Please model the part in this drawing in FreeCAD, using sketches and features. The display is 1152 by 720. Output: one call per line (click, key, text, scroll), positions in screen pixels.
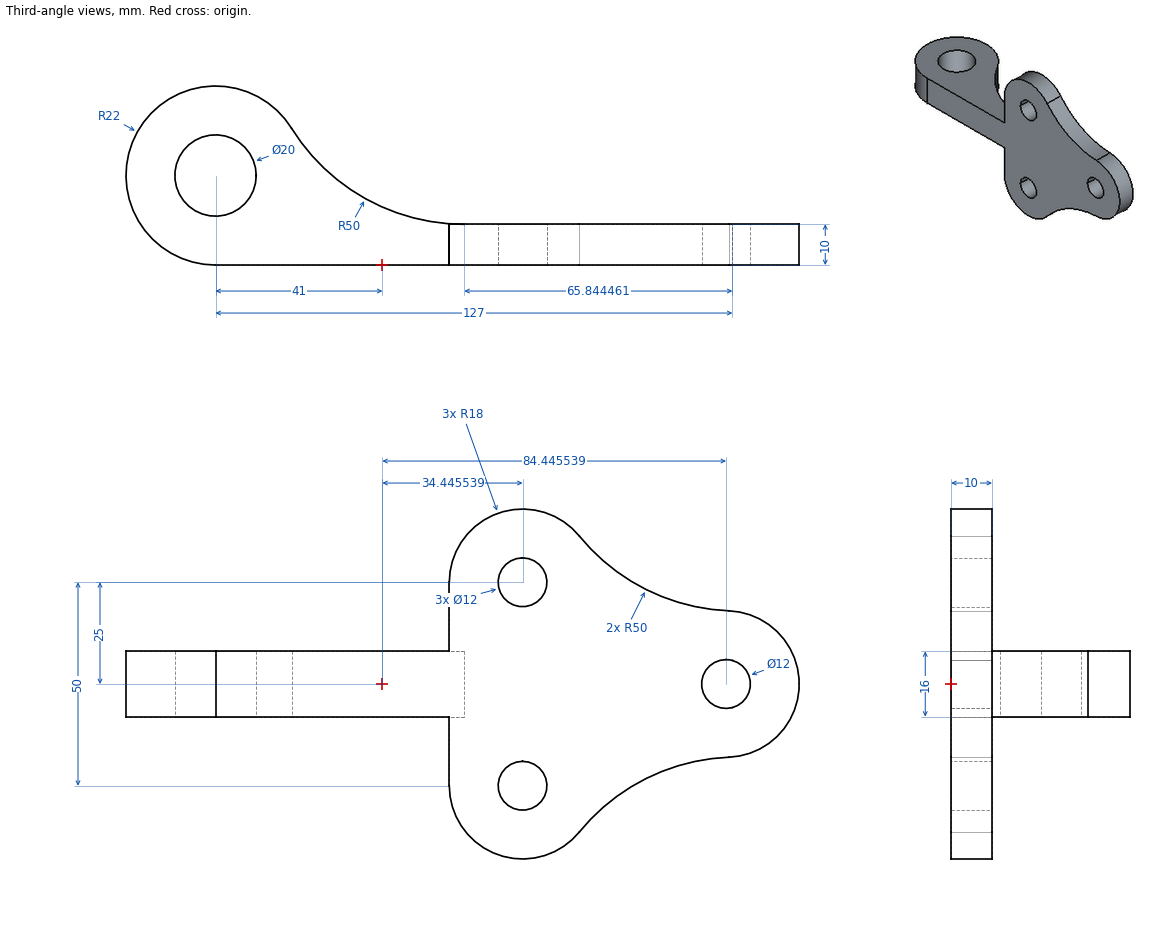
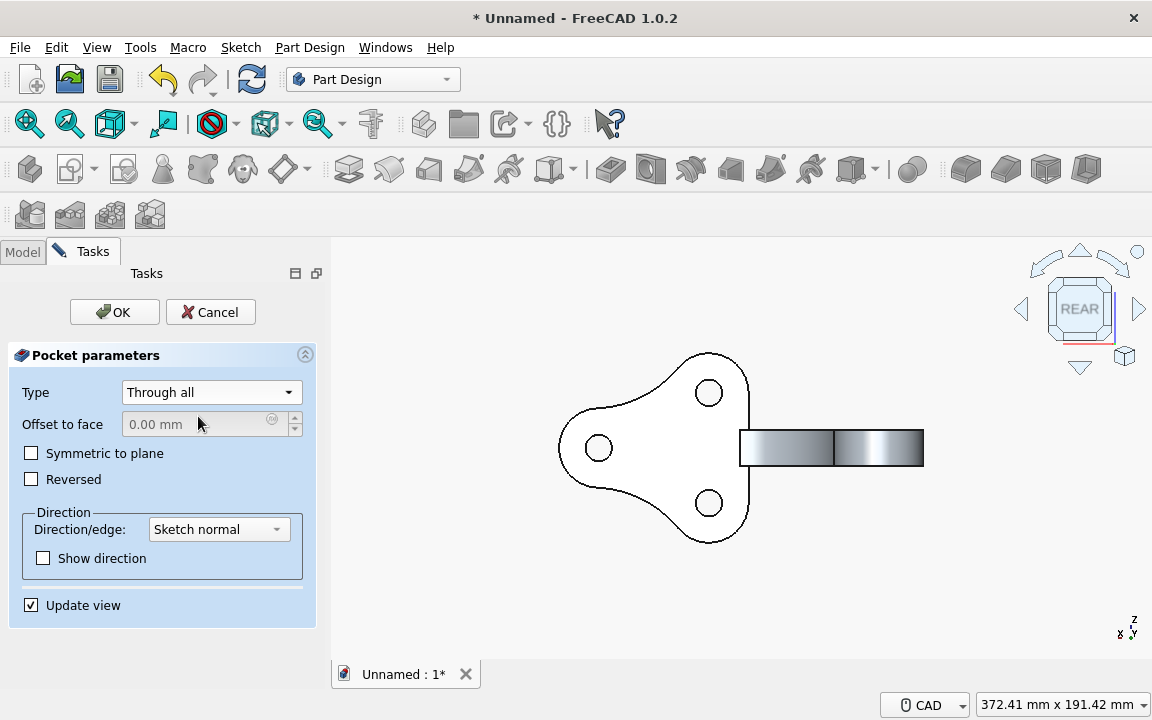
click(115, 312)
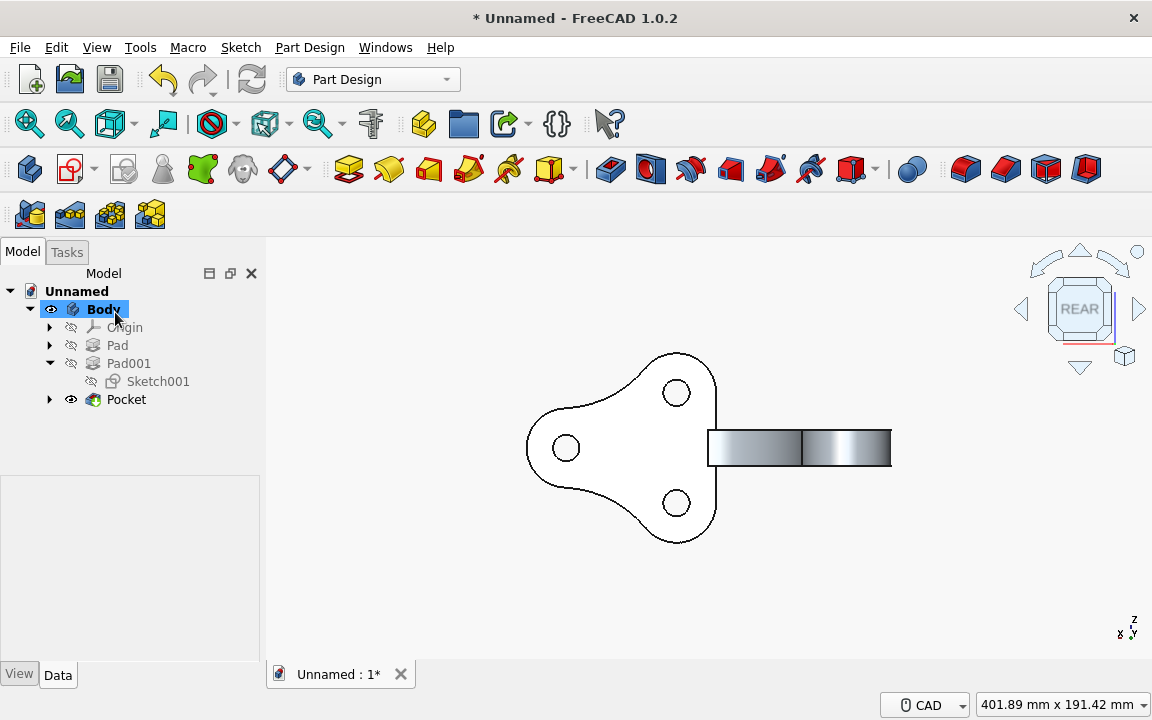
key(0)